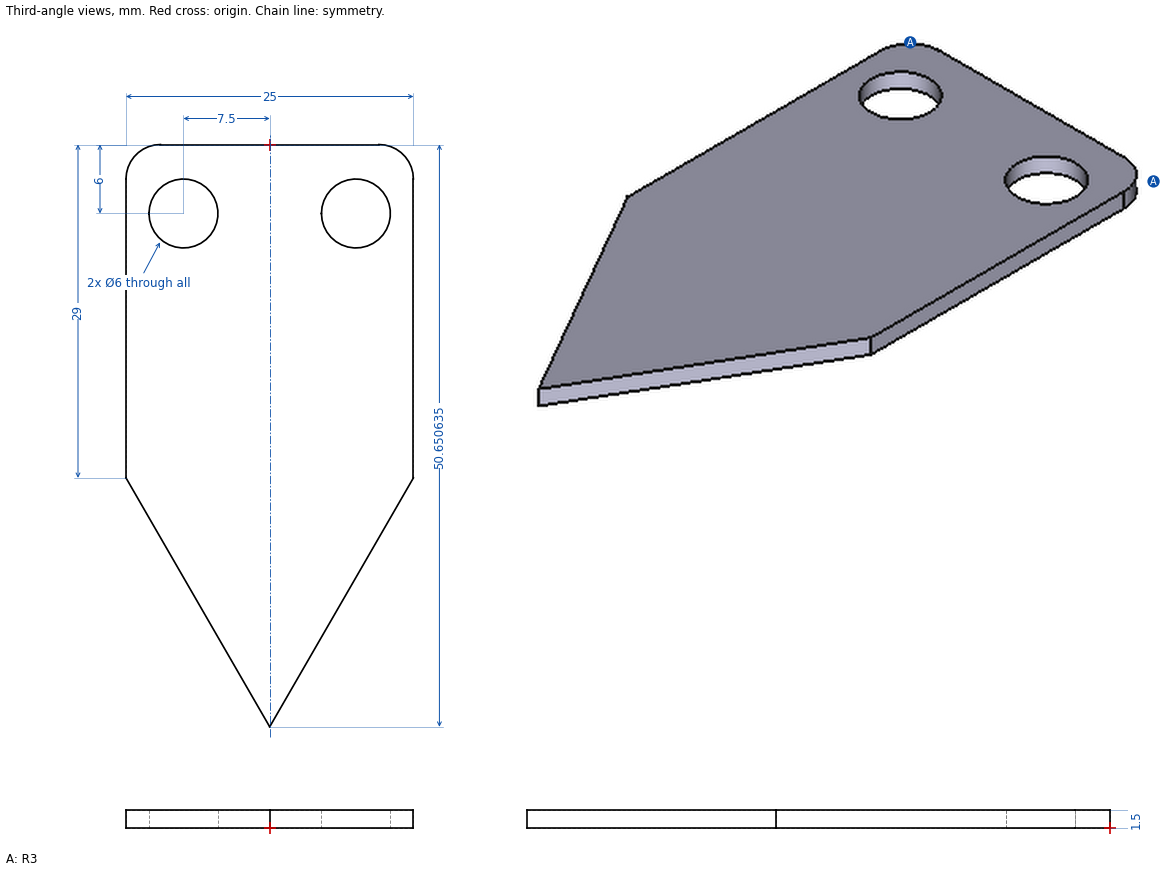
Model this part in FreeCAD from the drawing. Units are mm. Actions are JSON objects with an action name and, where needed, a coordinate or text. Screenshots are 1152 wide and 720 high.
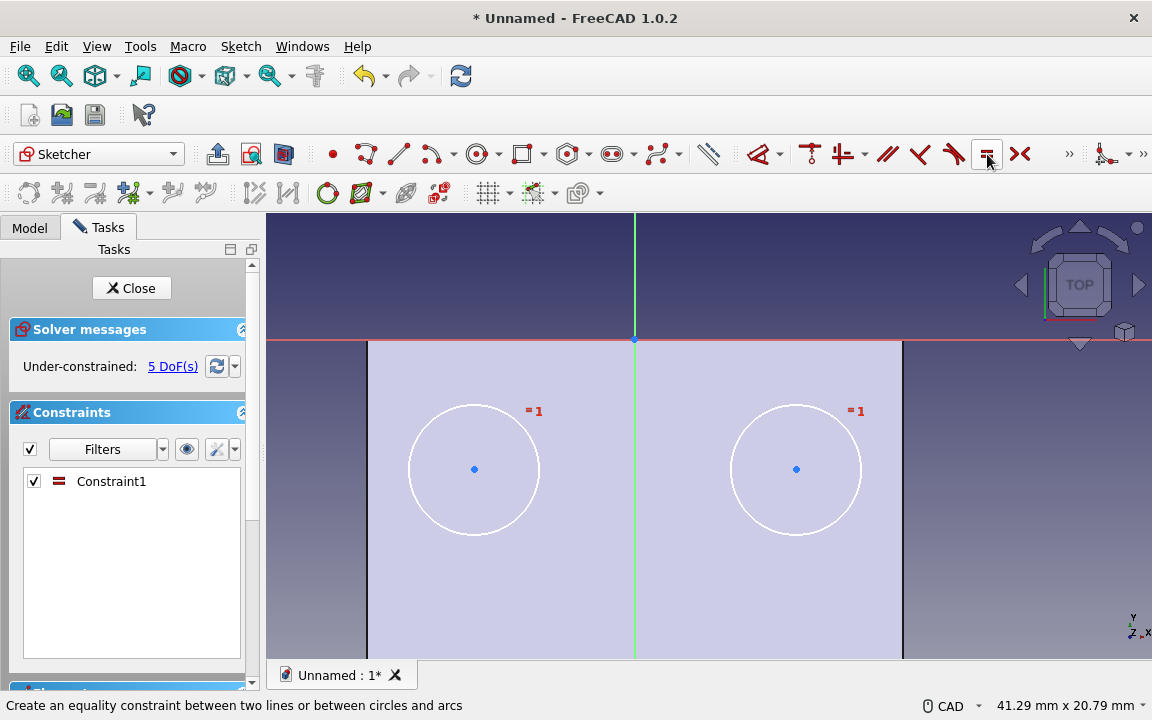
{"action": "left_click", "coordinate": [474, 470]}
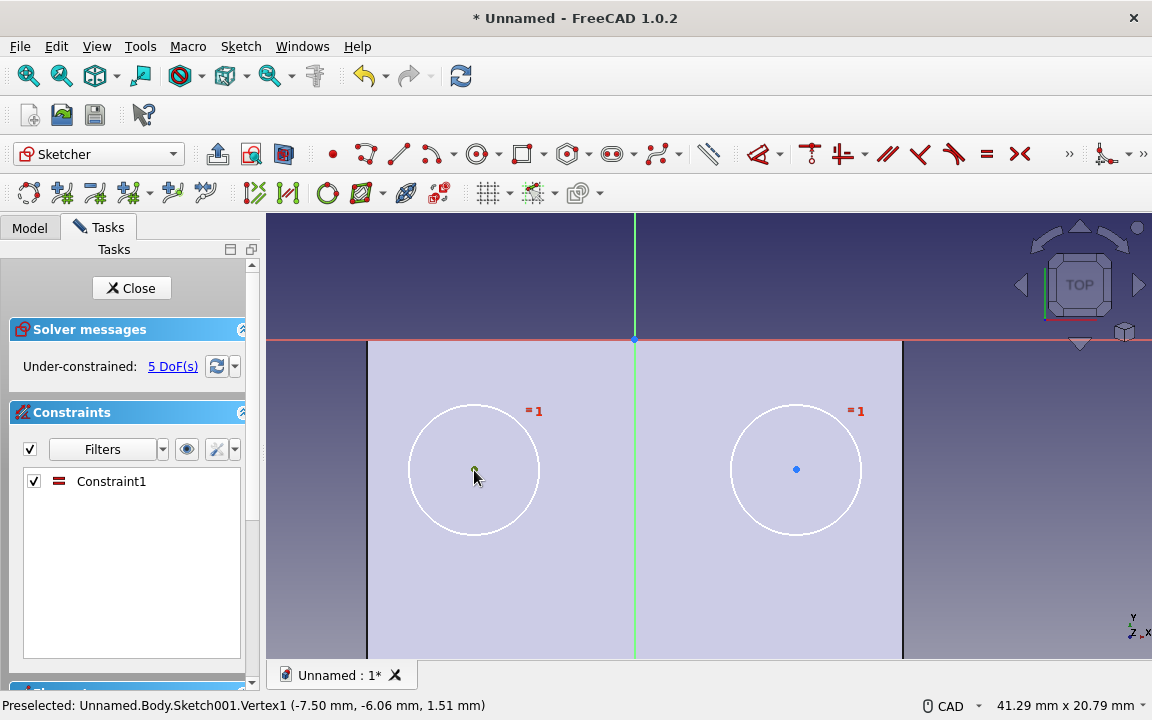
{"action": "left_click", "coordinate": [796, 470]}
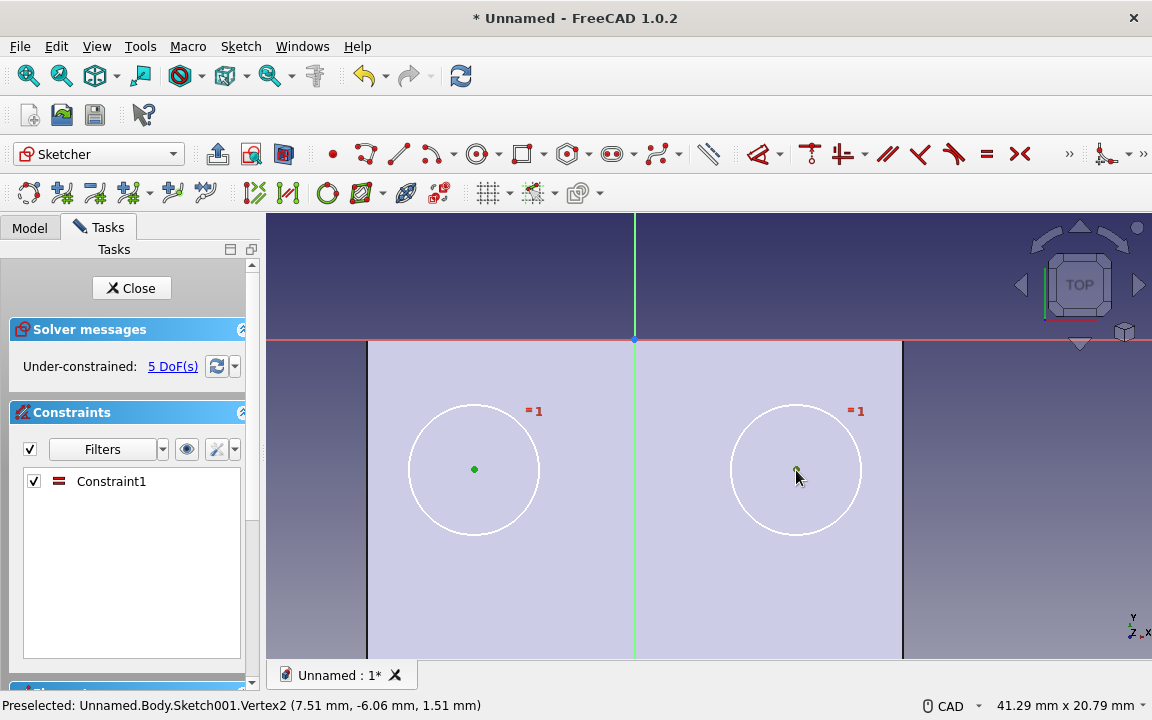
{"action": "left_click", "coordinate": [635, 603]}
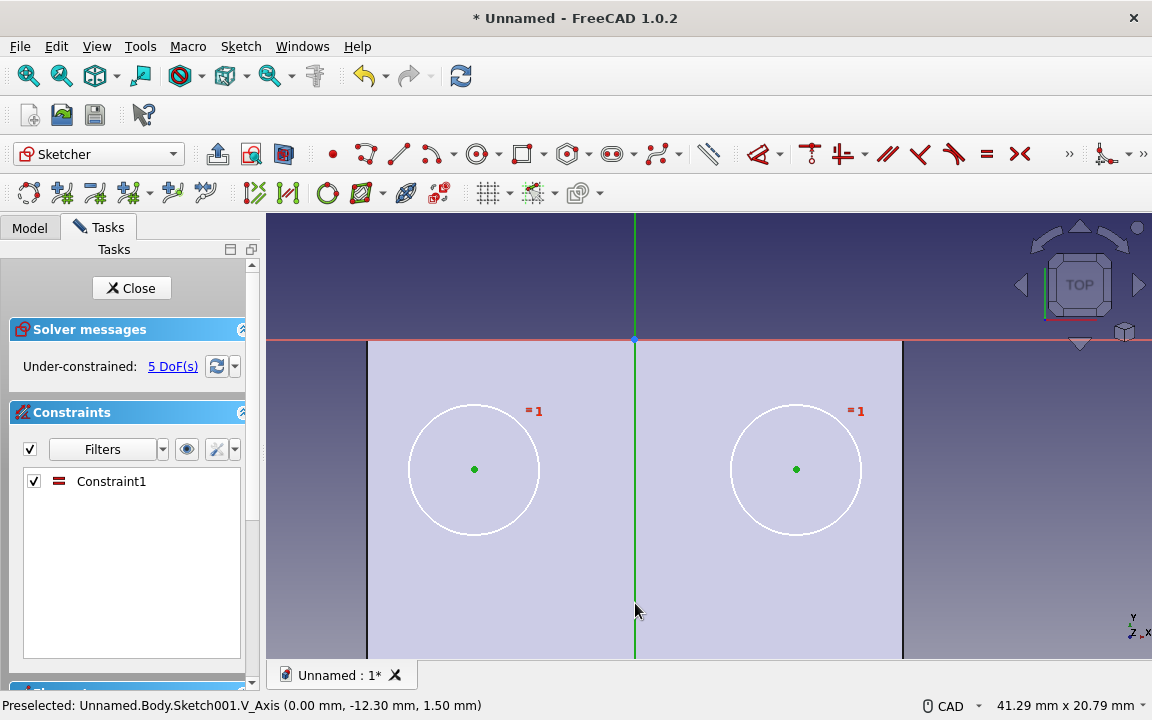
{"action": "left_click", "coordinate": [1020, 154]}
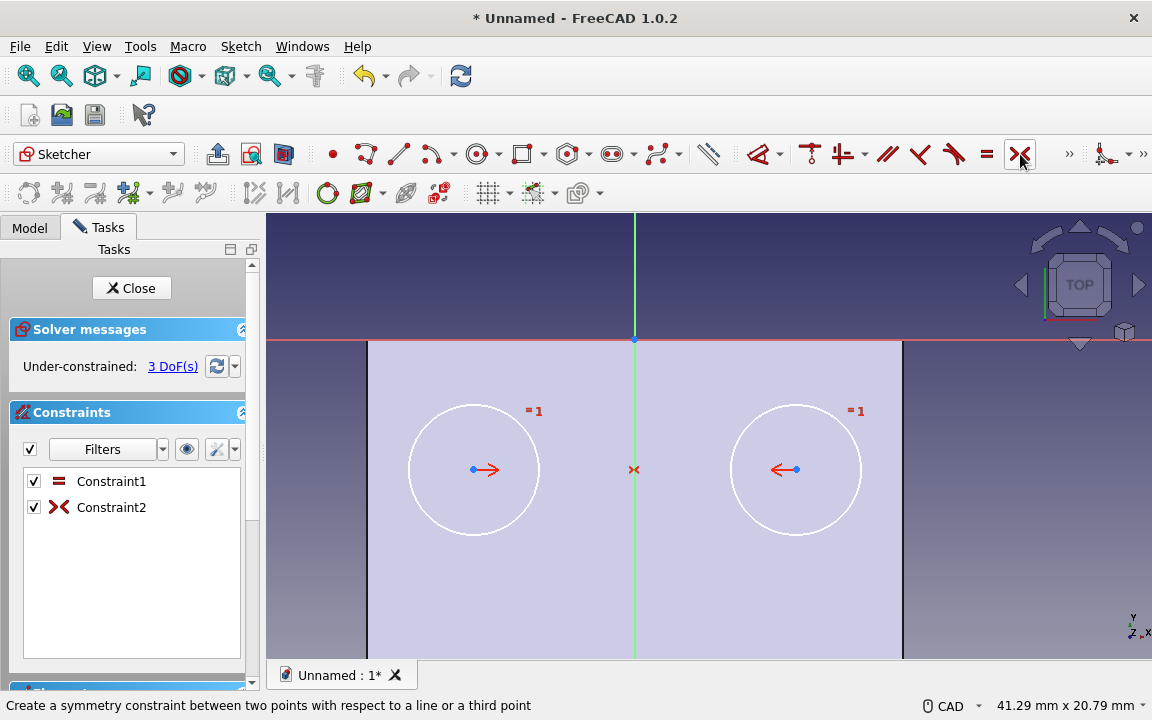
{"action": "left_click", "coordinate": [758, 154]}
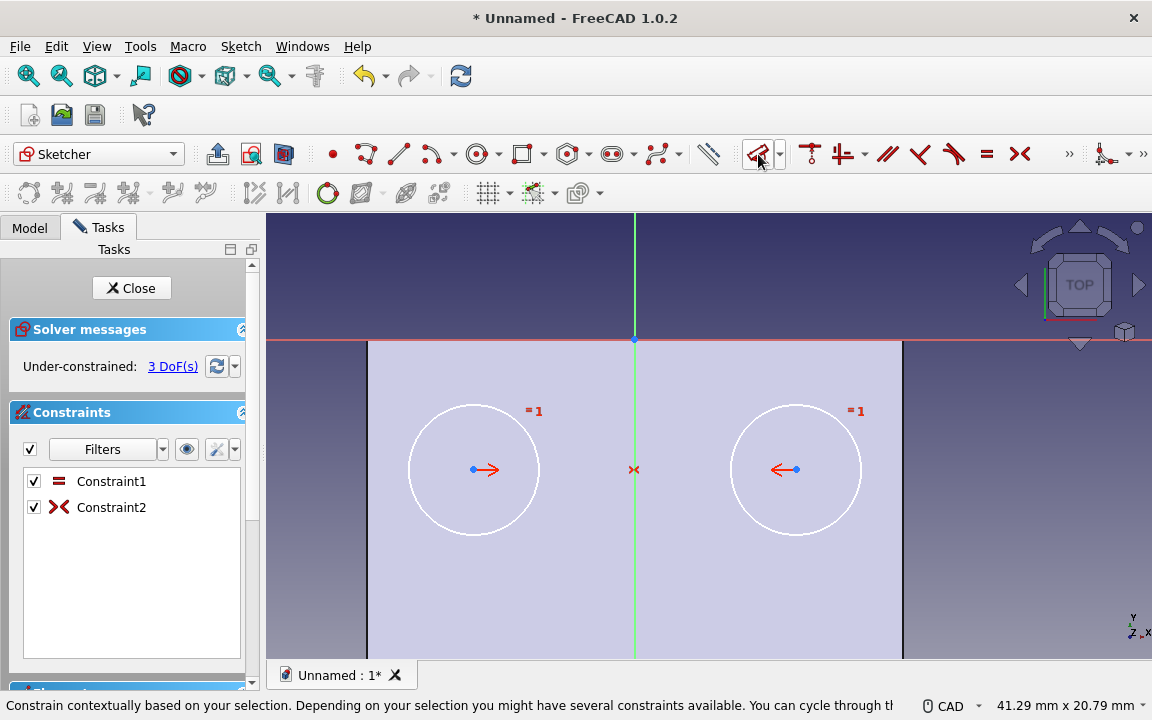
{"action": "left_click", "coordinate": [520, 424]}
{"action": "left_click", "coordinate": [543, 401]}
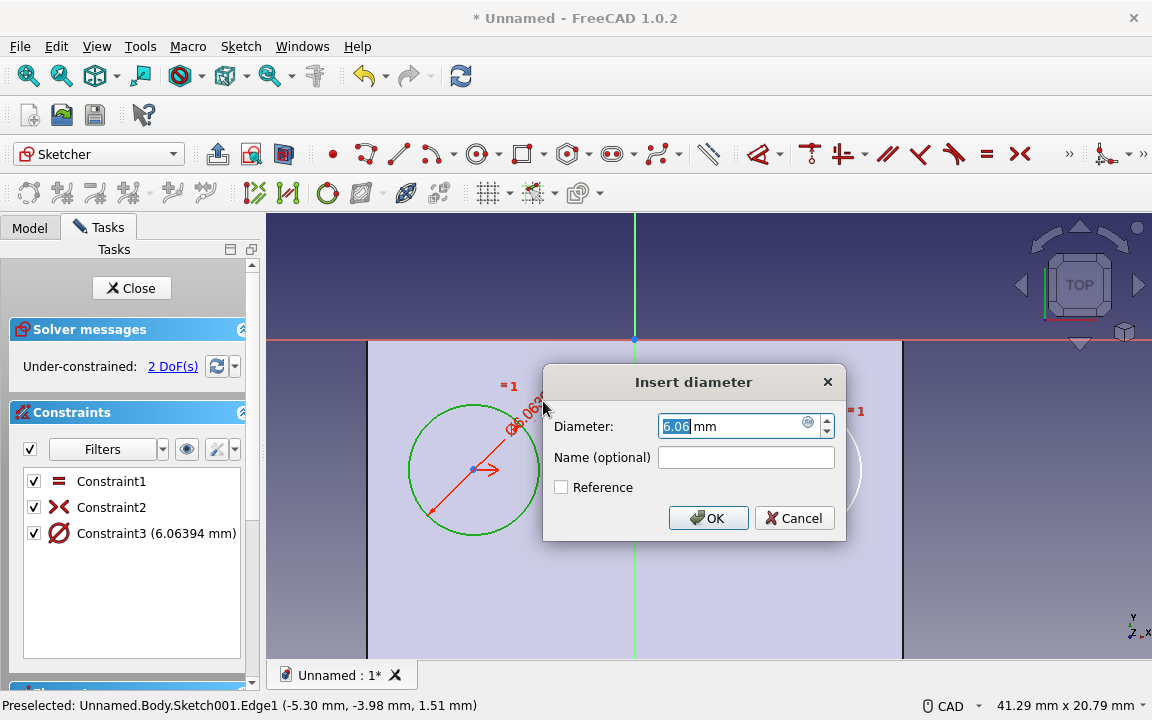
{"action": "type", "text": "6"}
{"action": "key", "text": "Return"}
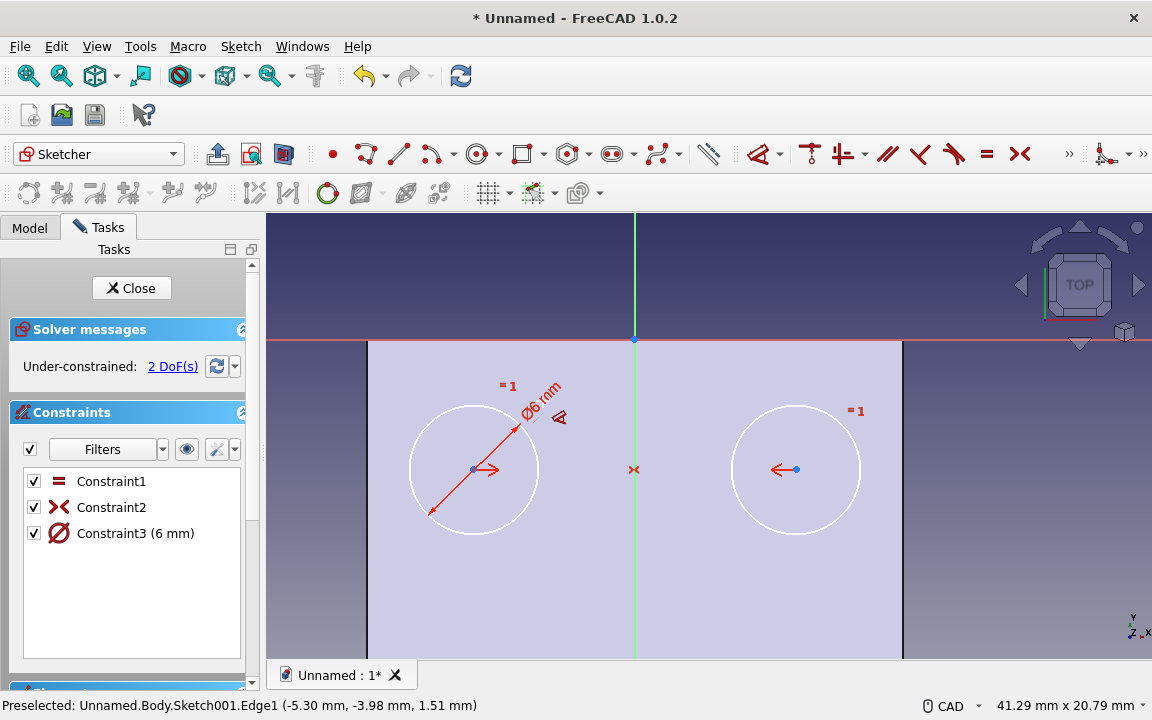
{"action": "left_click", "coordinate": [474, 470]}
{"action": "left_click", "coordinate": [440, 375]}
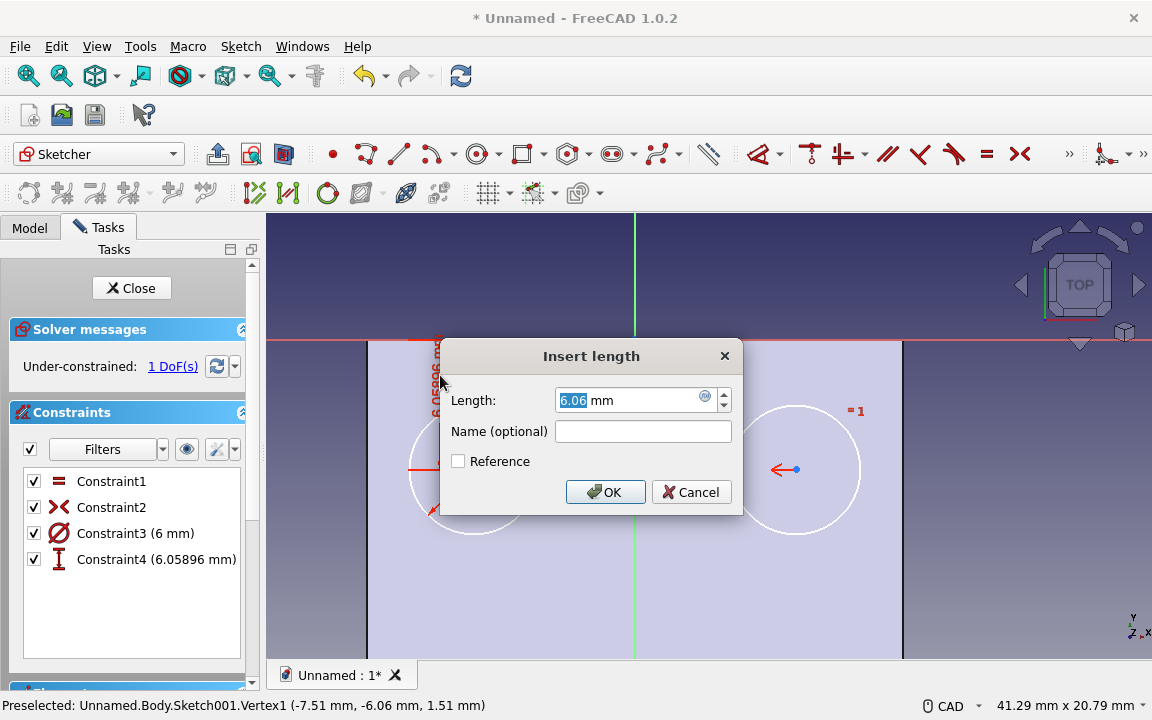
{"action": "type", "text": "6"}
{"action": "key", "text": "Return"}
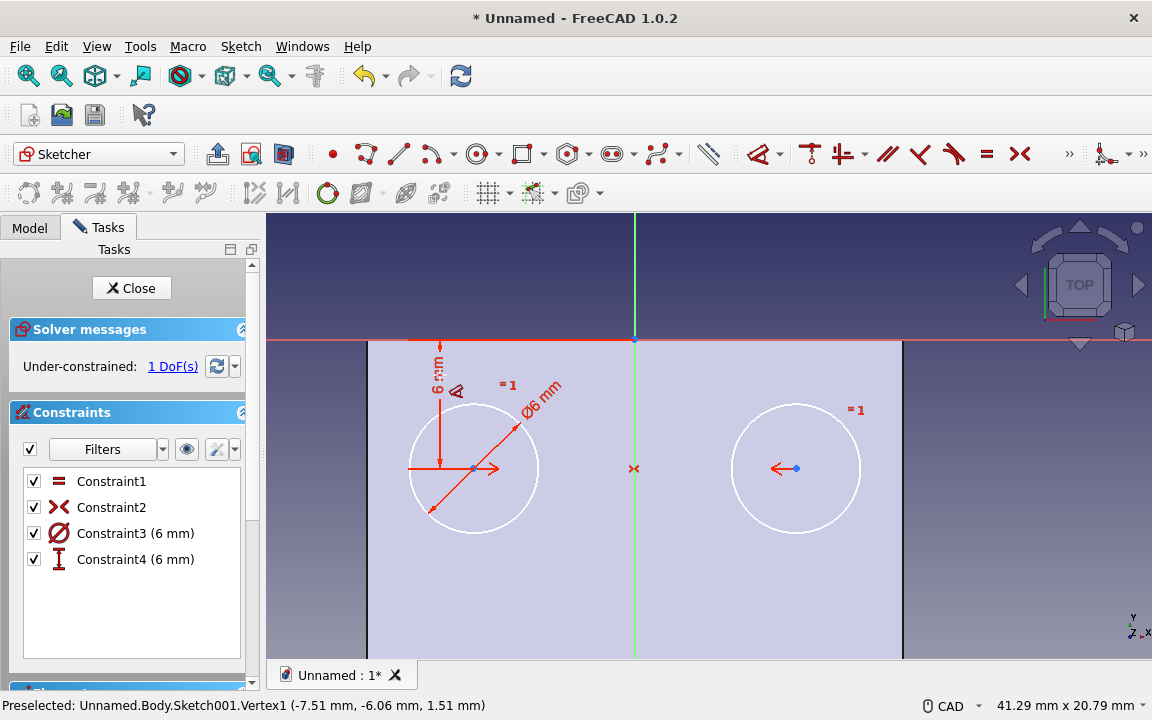
{"action": "left_click", "coordinate": [474, 469]}
{"action": "left_click", "coordinate": [554, 306]}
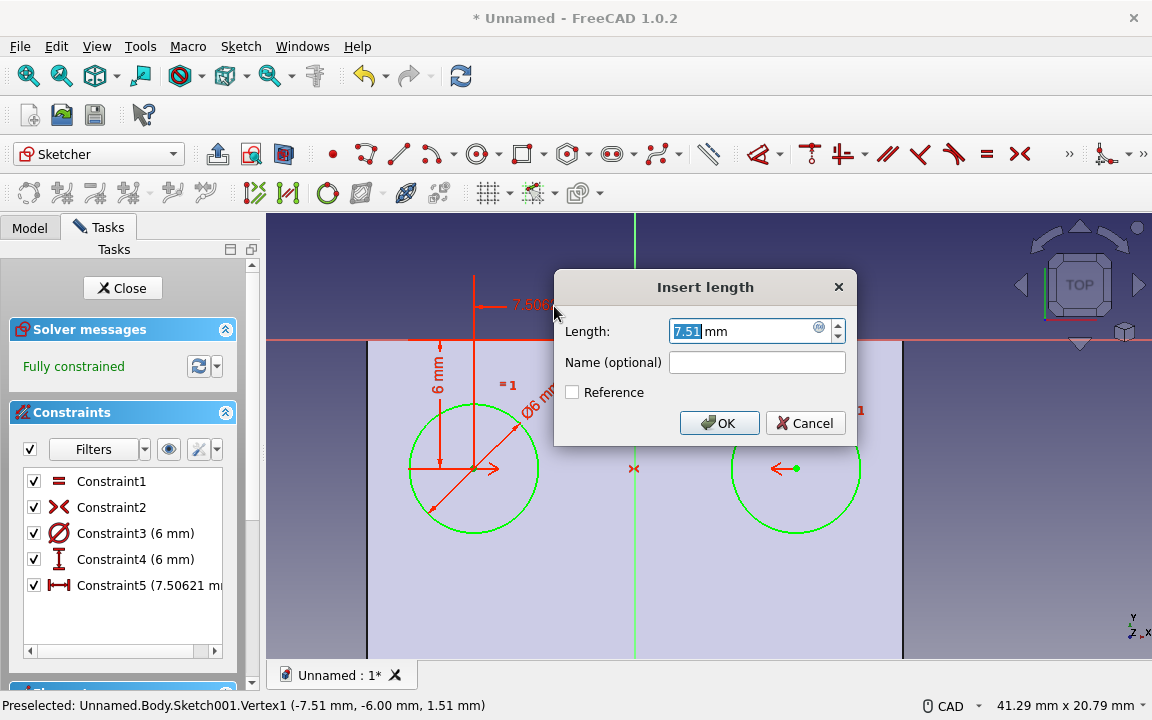
{"action": "type", "text": "7.5"}
{"action": "key", "text": "Return"}
{"action": "key", "text": "Escape"}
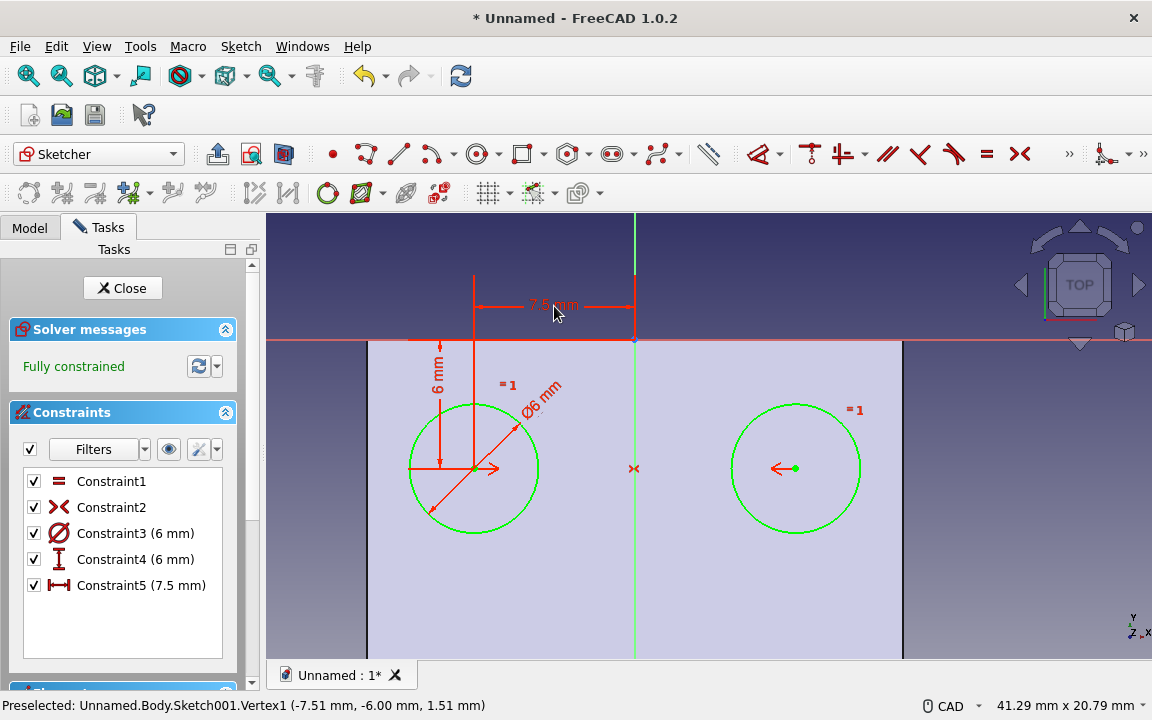
{"action": "left_click", "coordinate": [123, 288]}